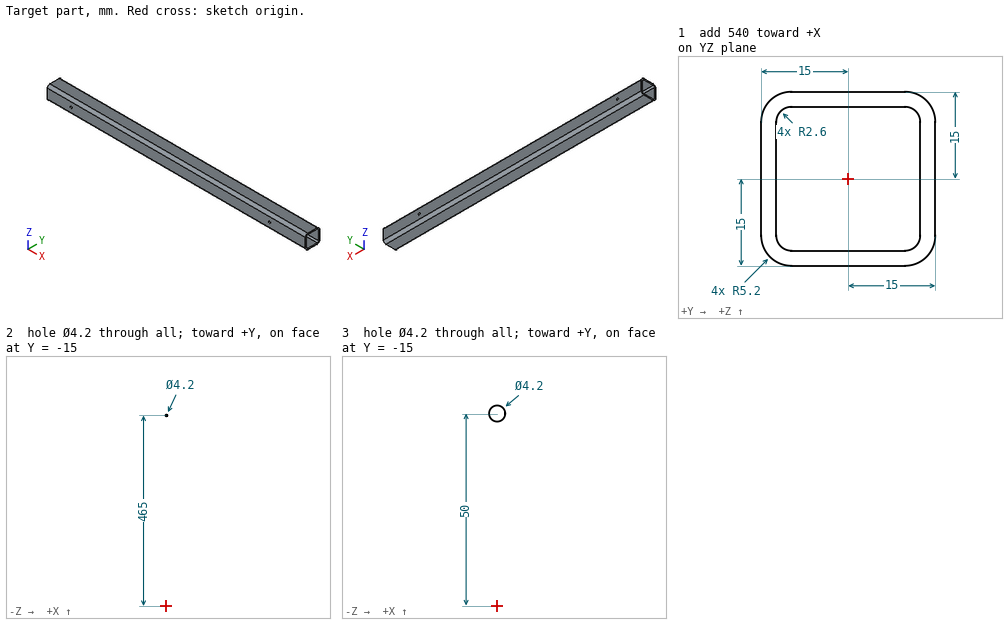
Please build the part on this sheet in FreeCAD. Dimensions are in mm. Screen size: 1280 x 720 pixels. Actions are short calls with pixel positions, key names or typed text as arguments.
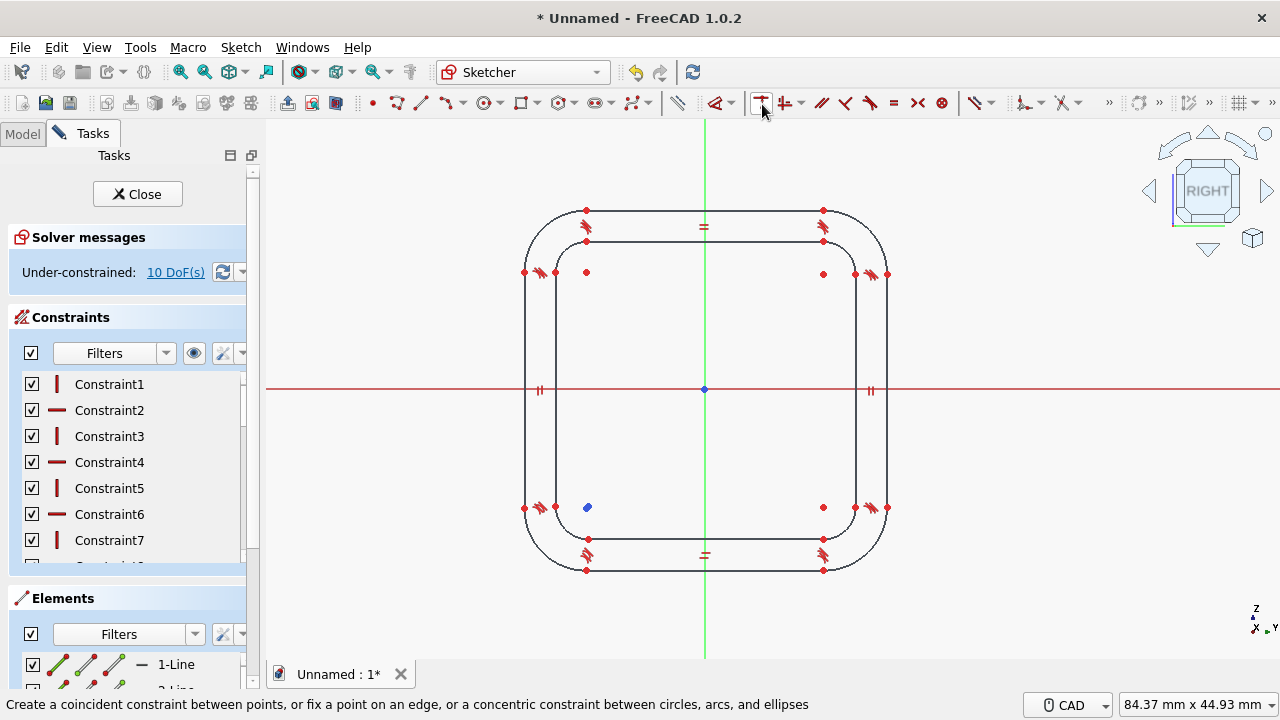
click(531, 537)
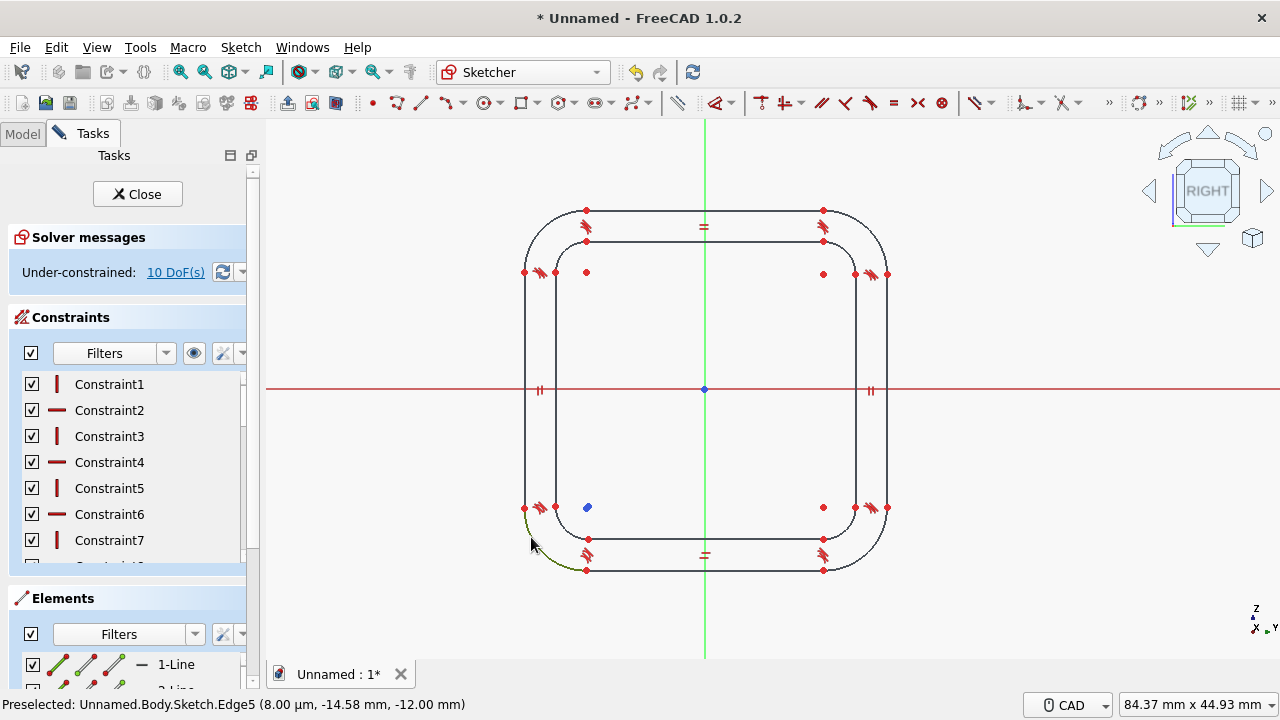
click(852, 564)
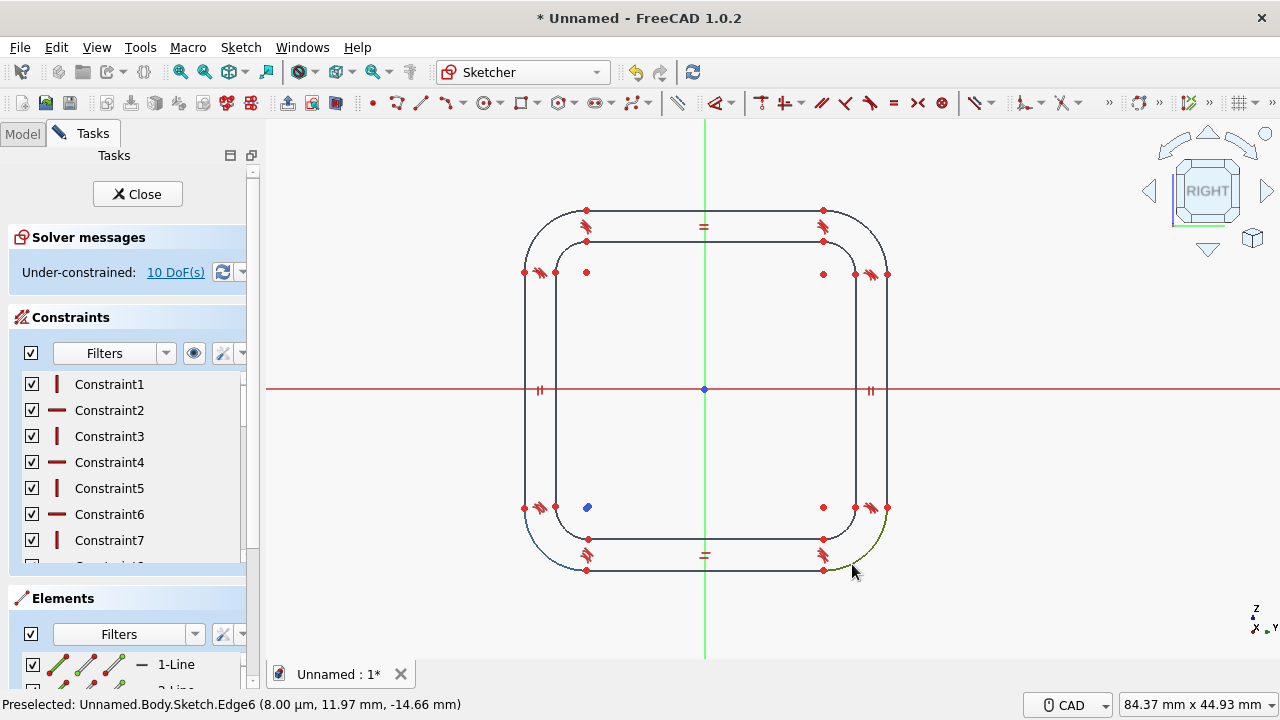
click(880, 245)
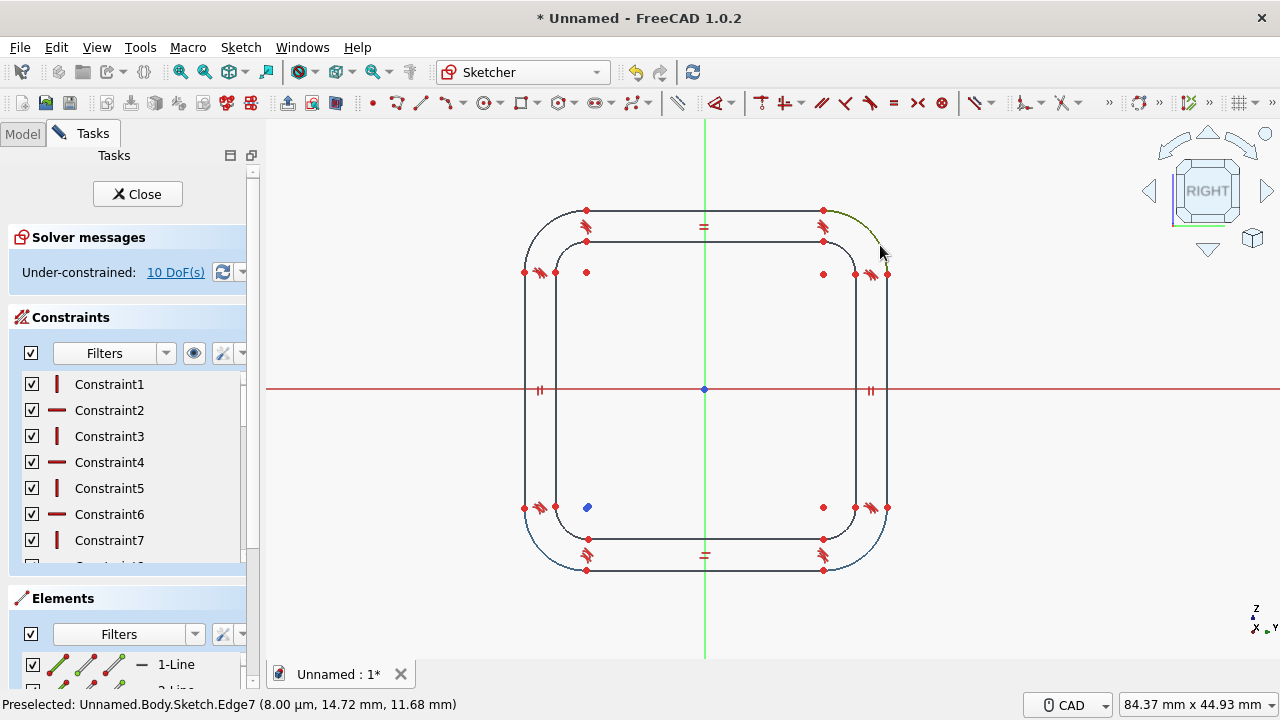
click(558, 217)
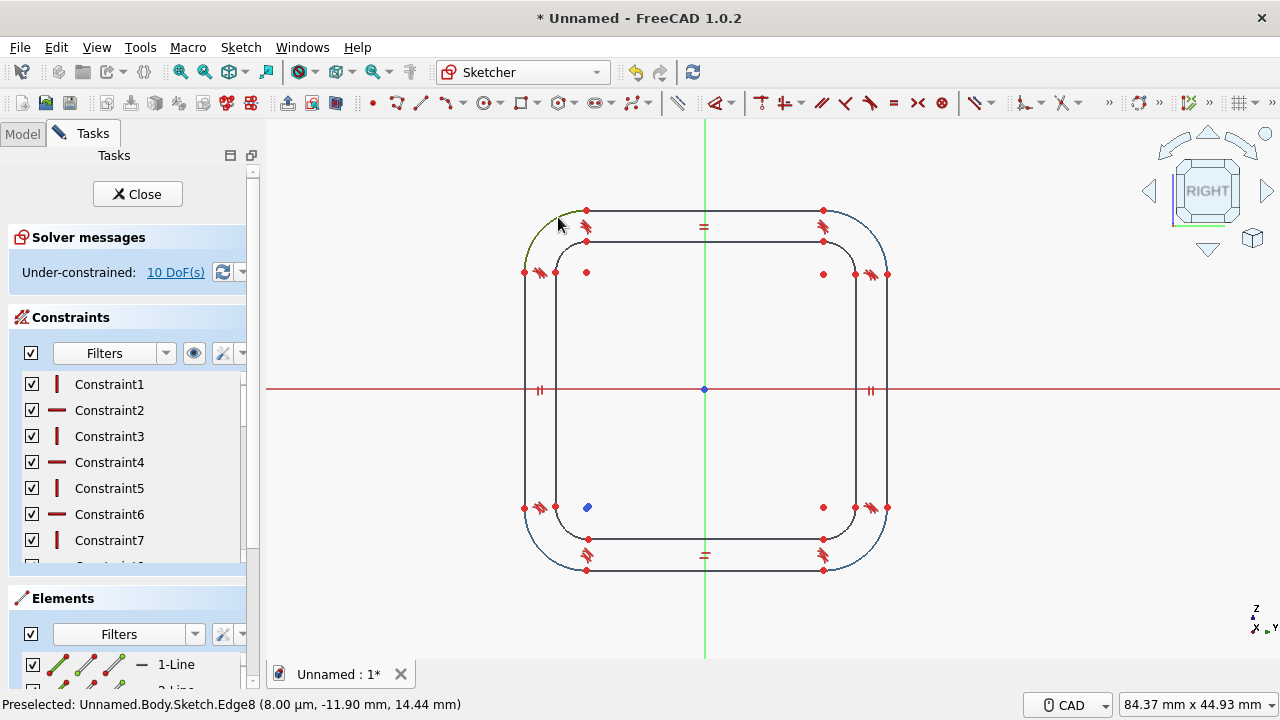
click(894, 104)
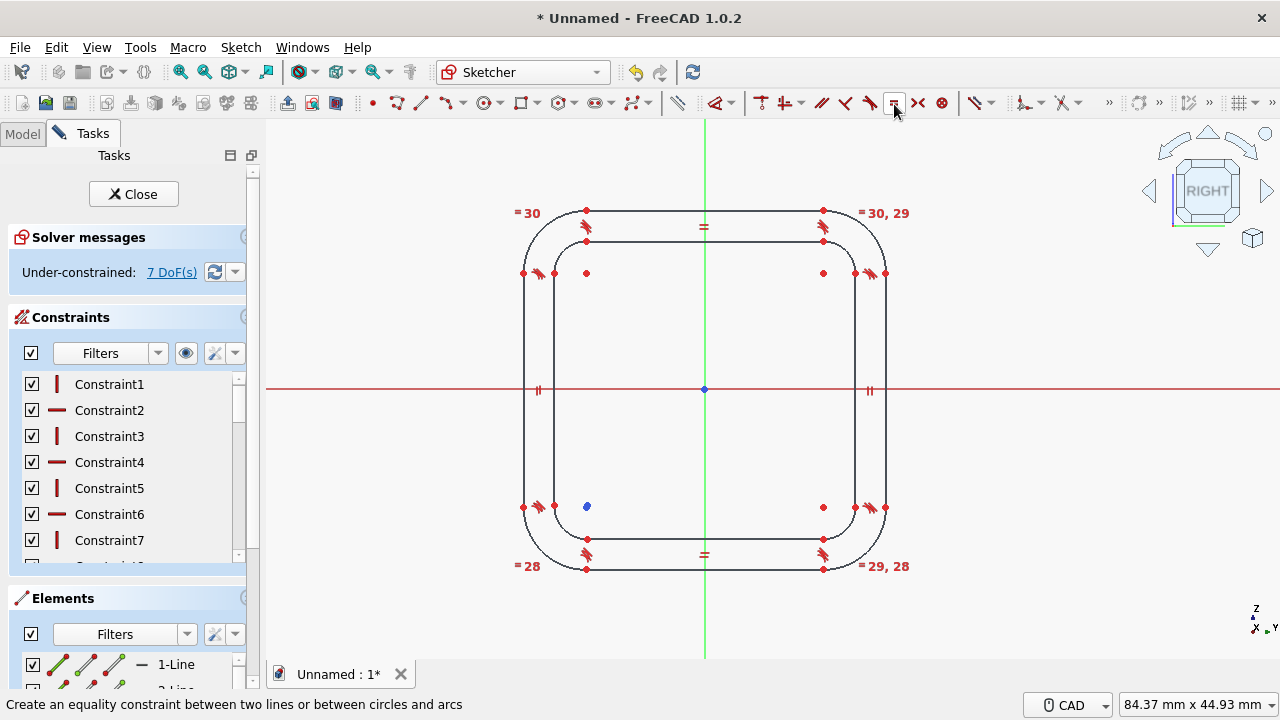
click(572, 245)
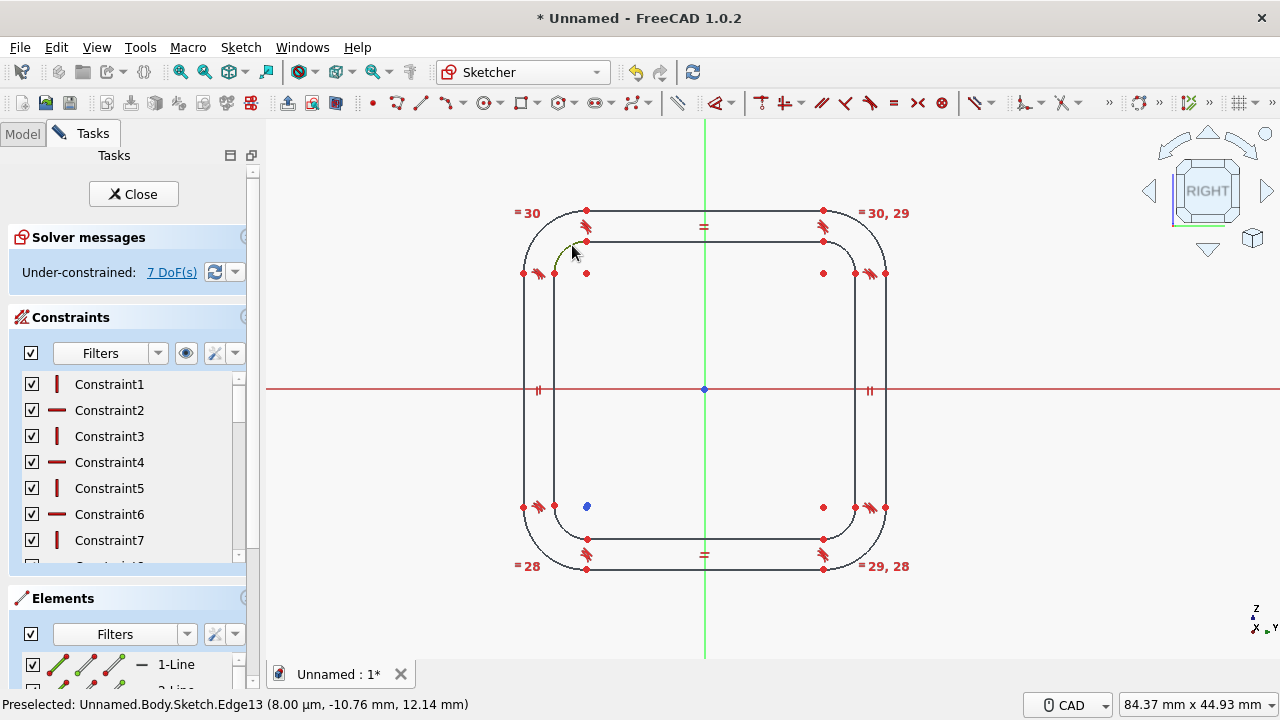
click(558, 521)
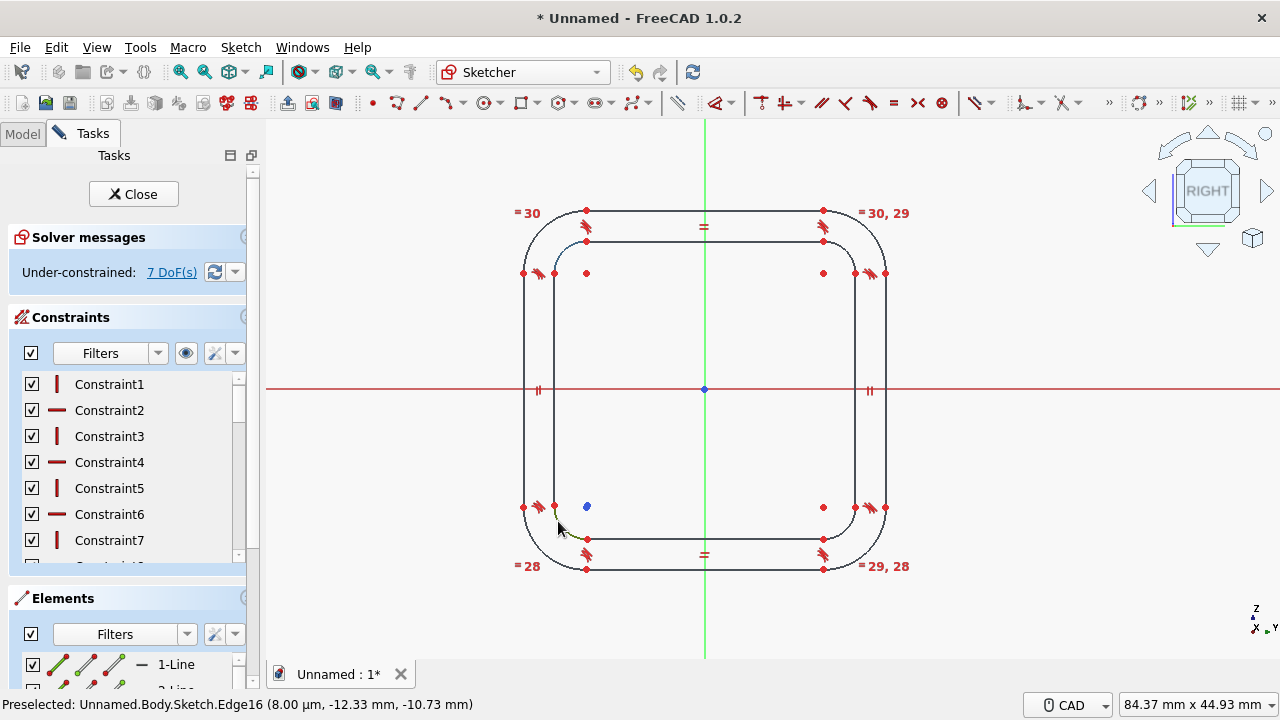
click(894, 104)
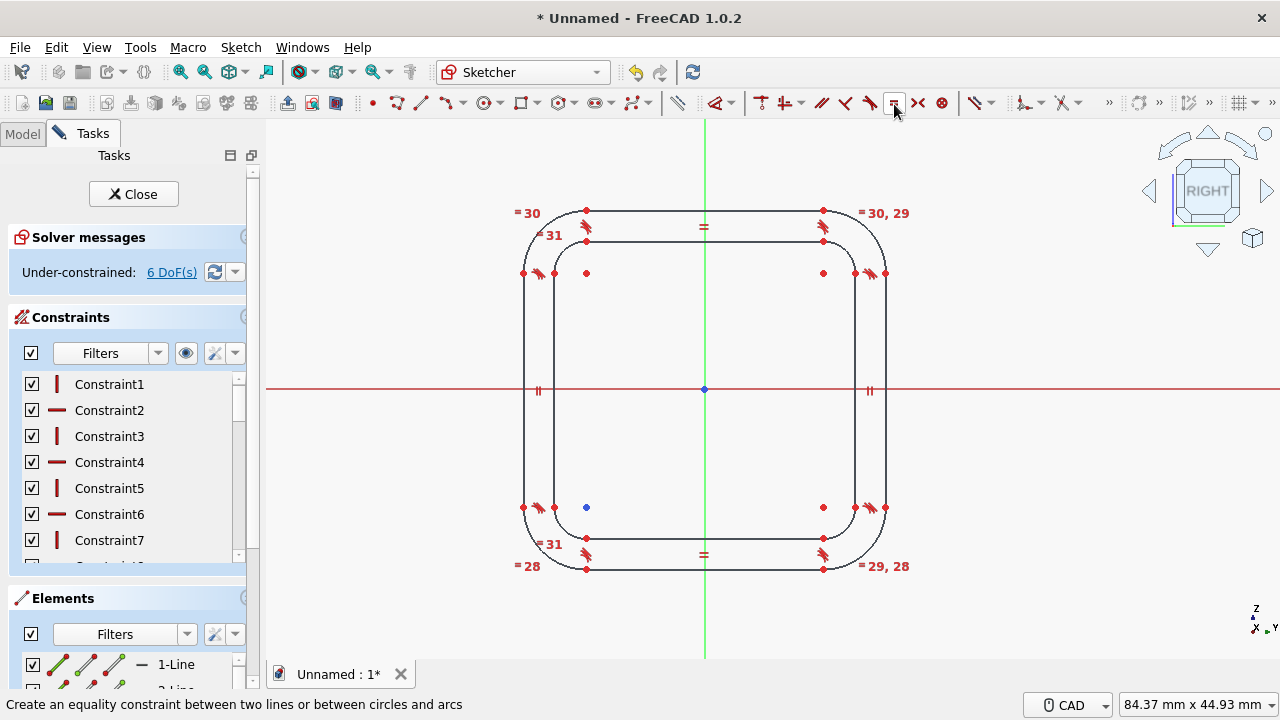
key(d)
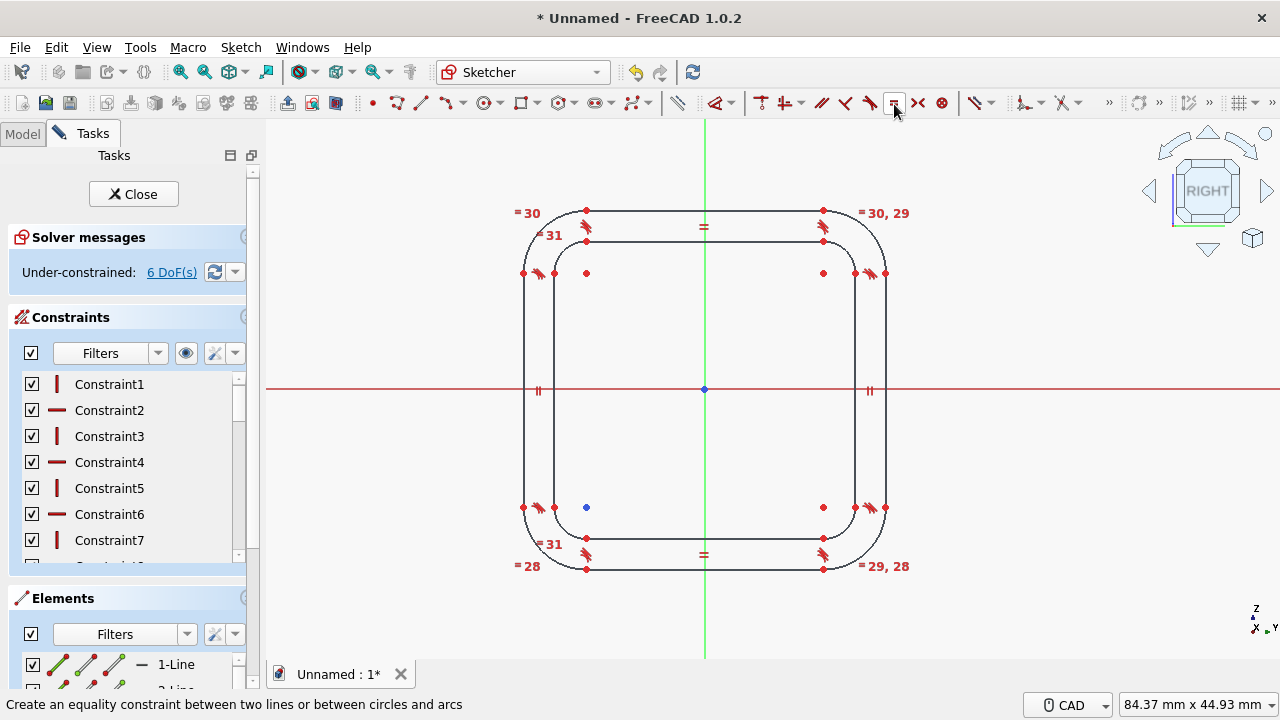
click(531, 535)
click(502, 549)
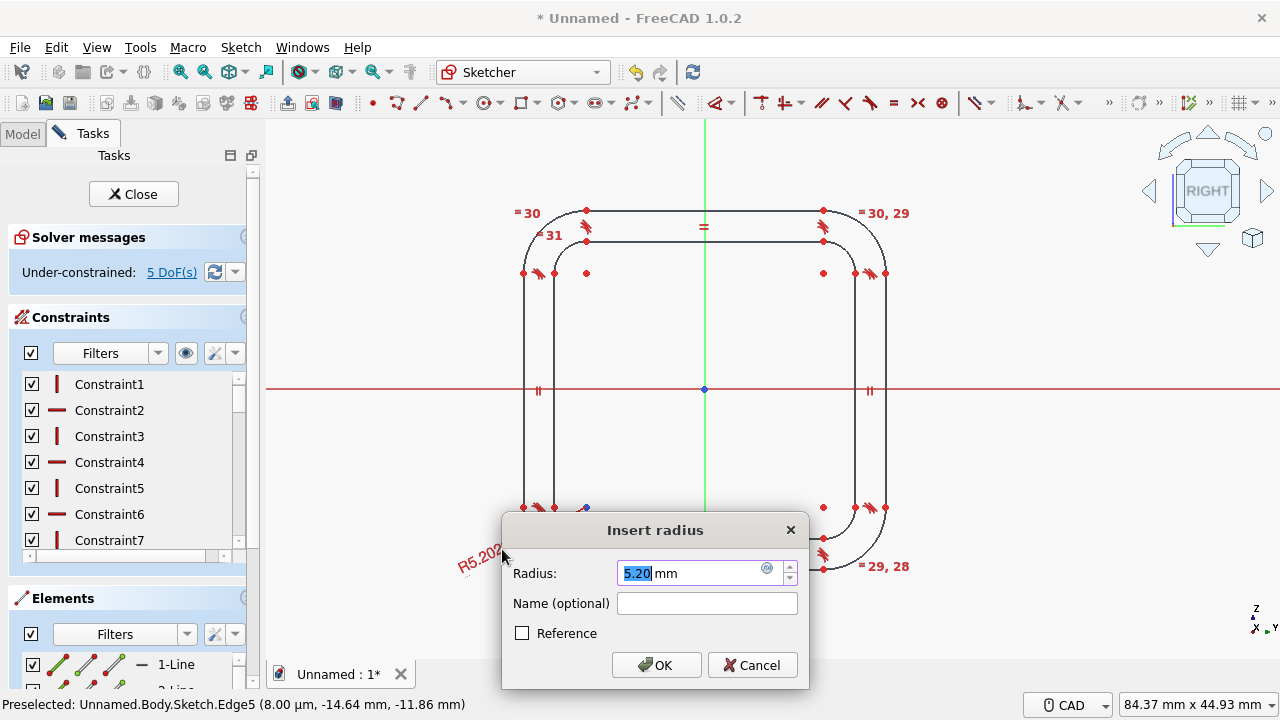
text(5.2)
key(Return)